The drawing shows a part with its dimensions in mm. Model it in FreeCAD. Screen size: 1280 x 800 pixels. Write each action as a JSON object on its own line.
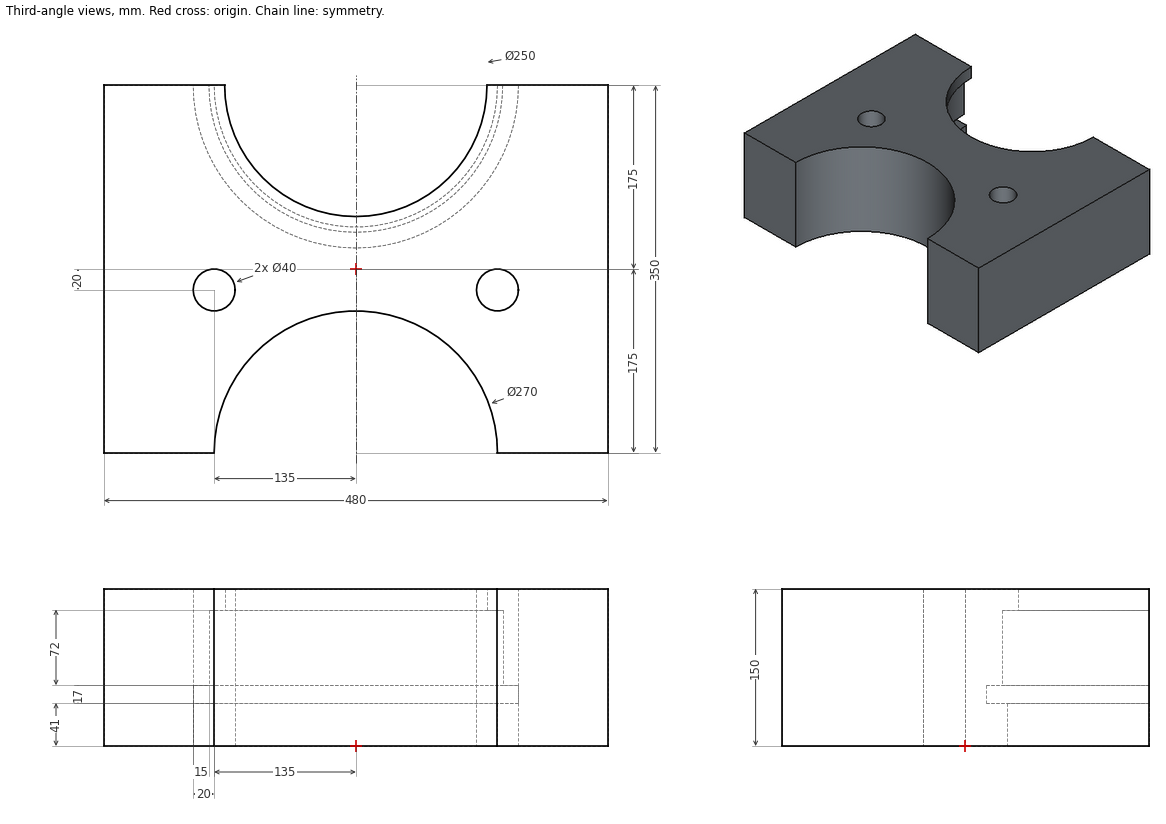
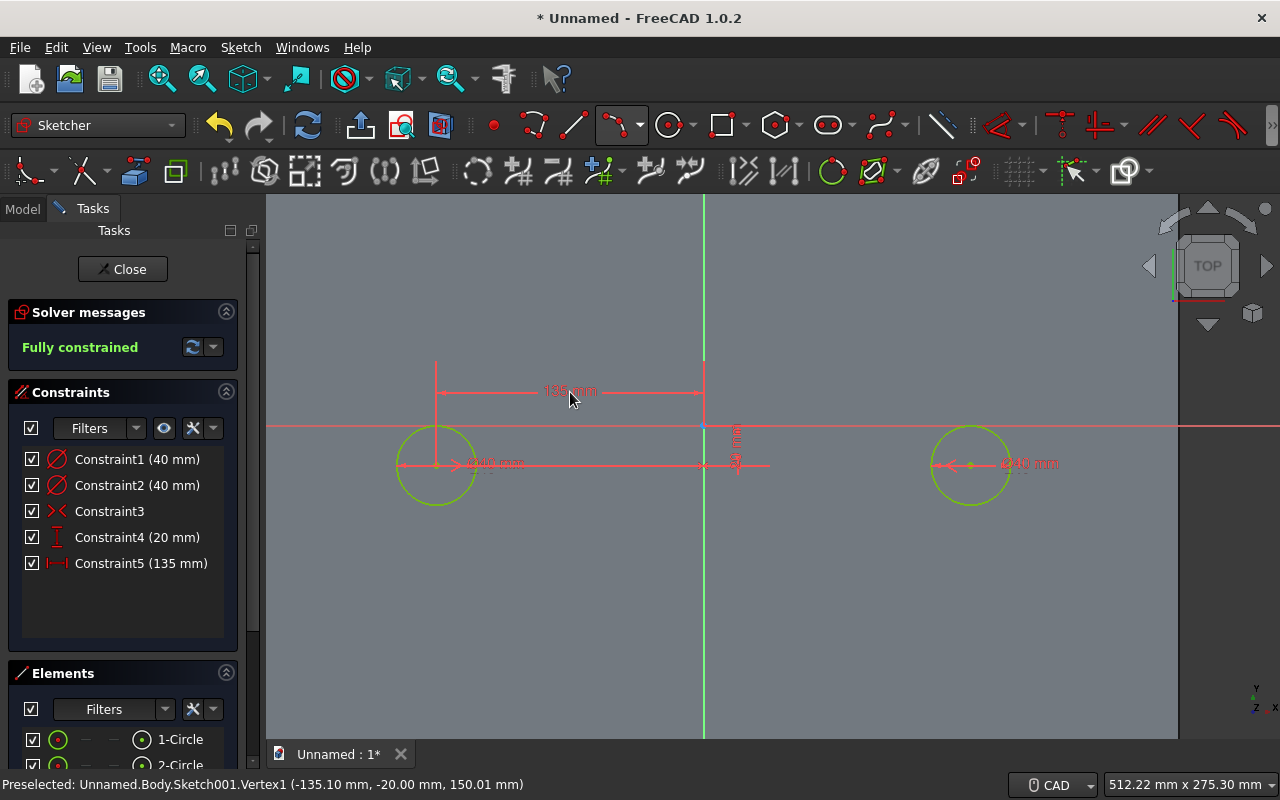
{"action": "left_click", "coordinate": [123, 269]}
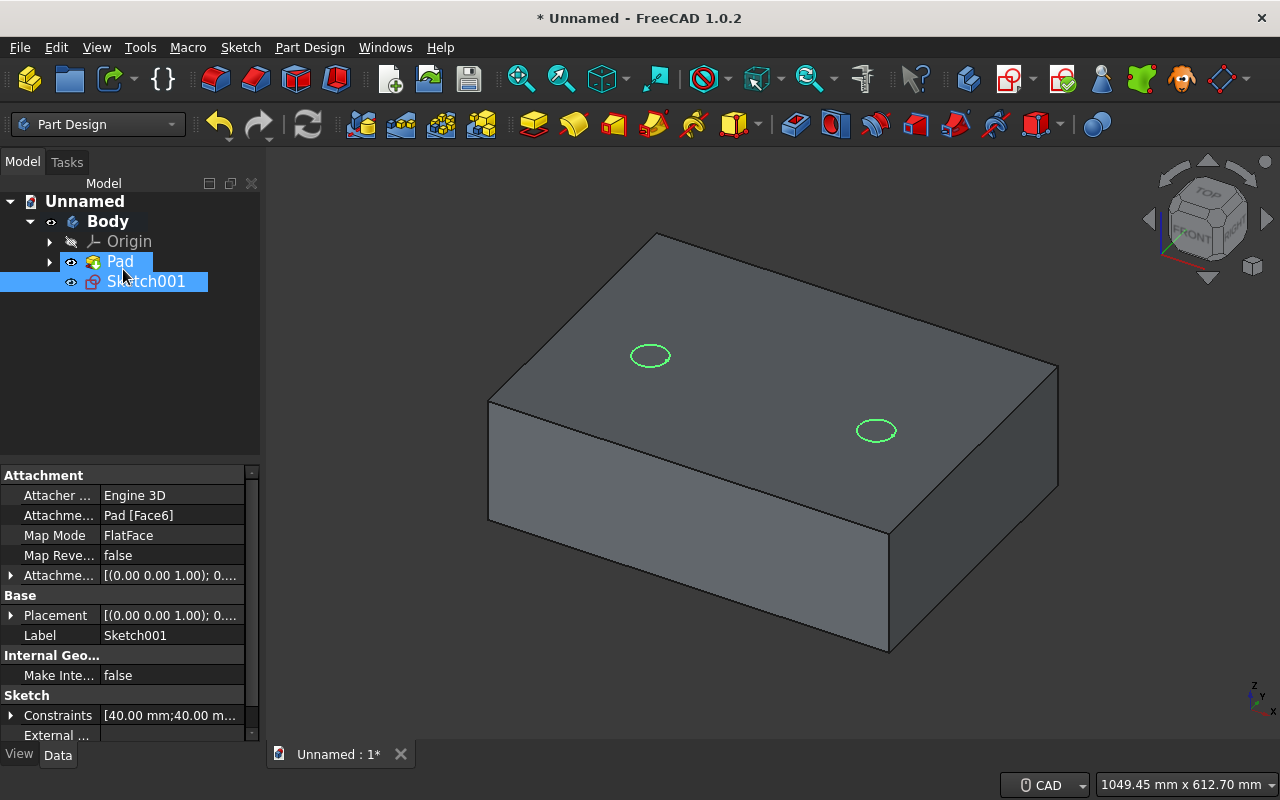
{"action": "left_click", "coordinate": [796, 124]}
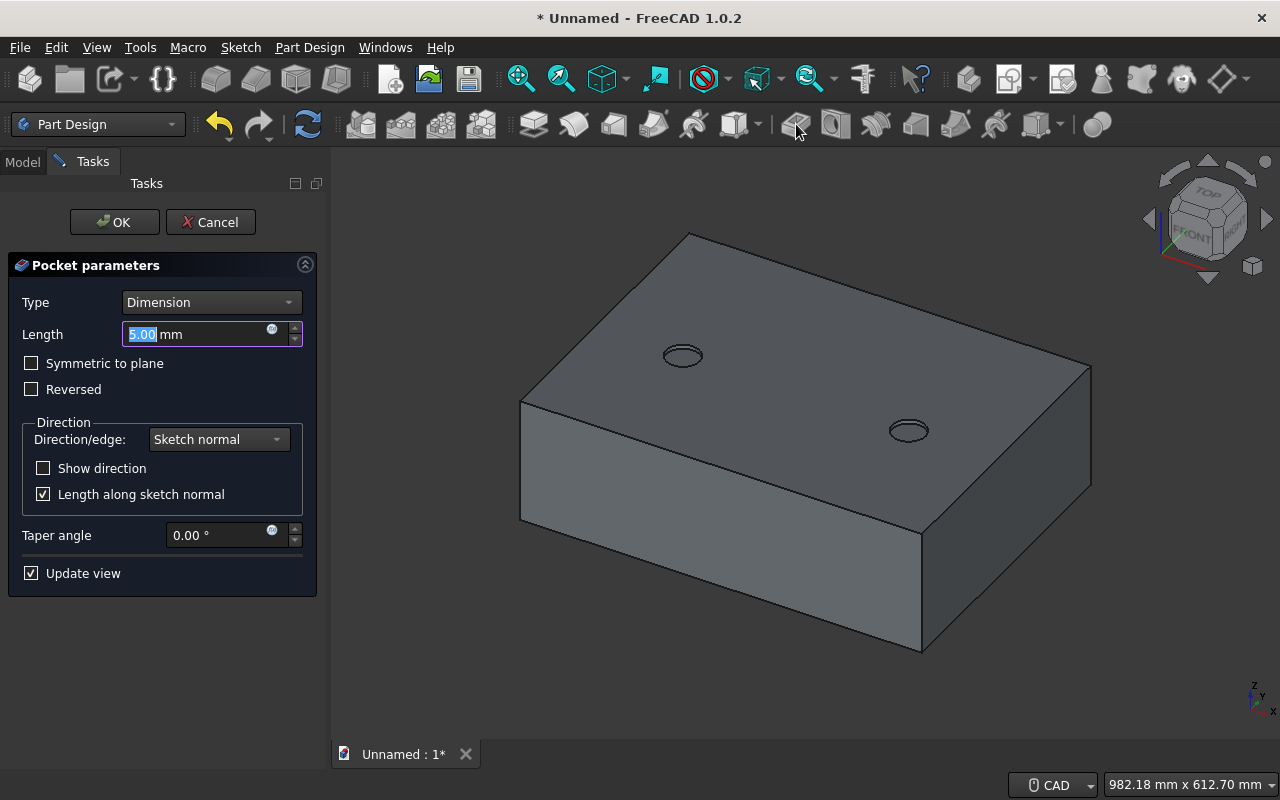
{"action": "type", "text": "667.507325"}
{"action": "key", "text": "Tab"}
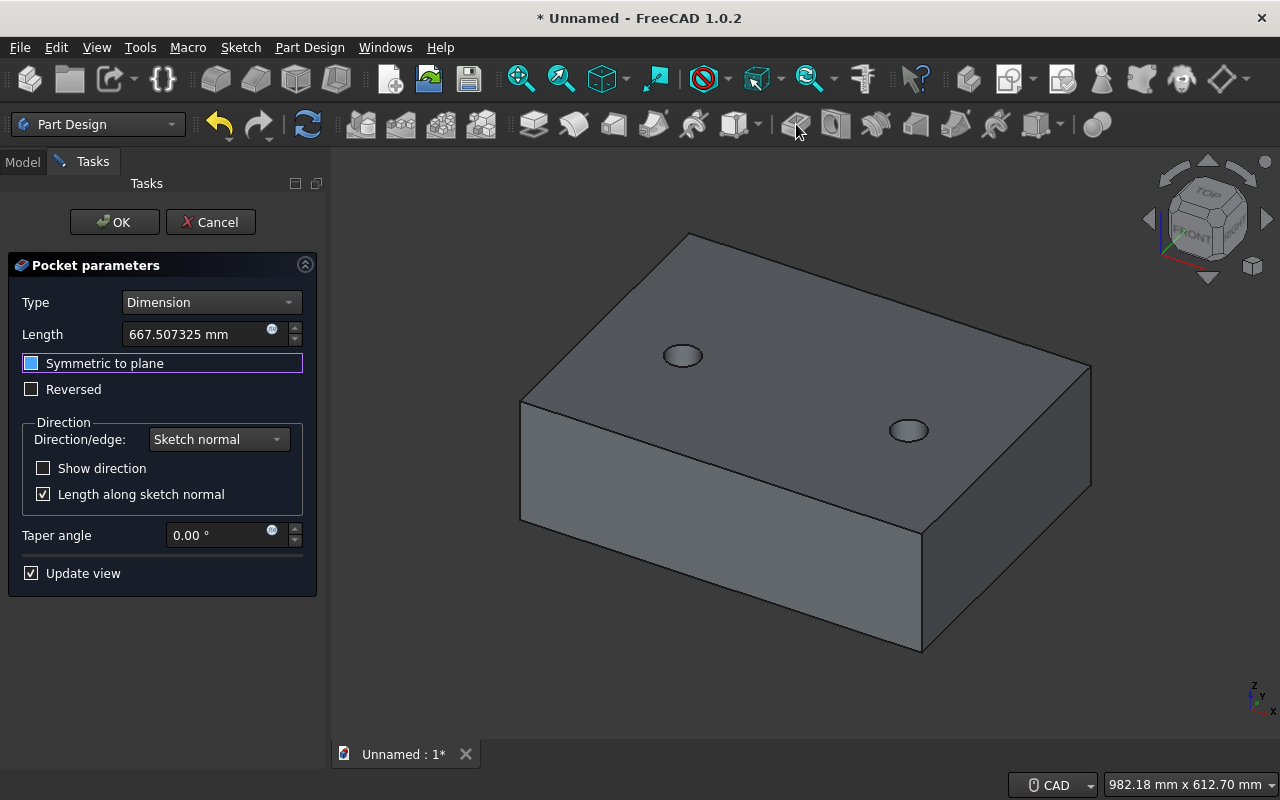
{"action": "left_click", "coordinate": [30, 363]}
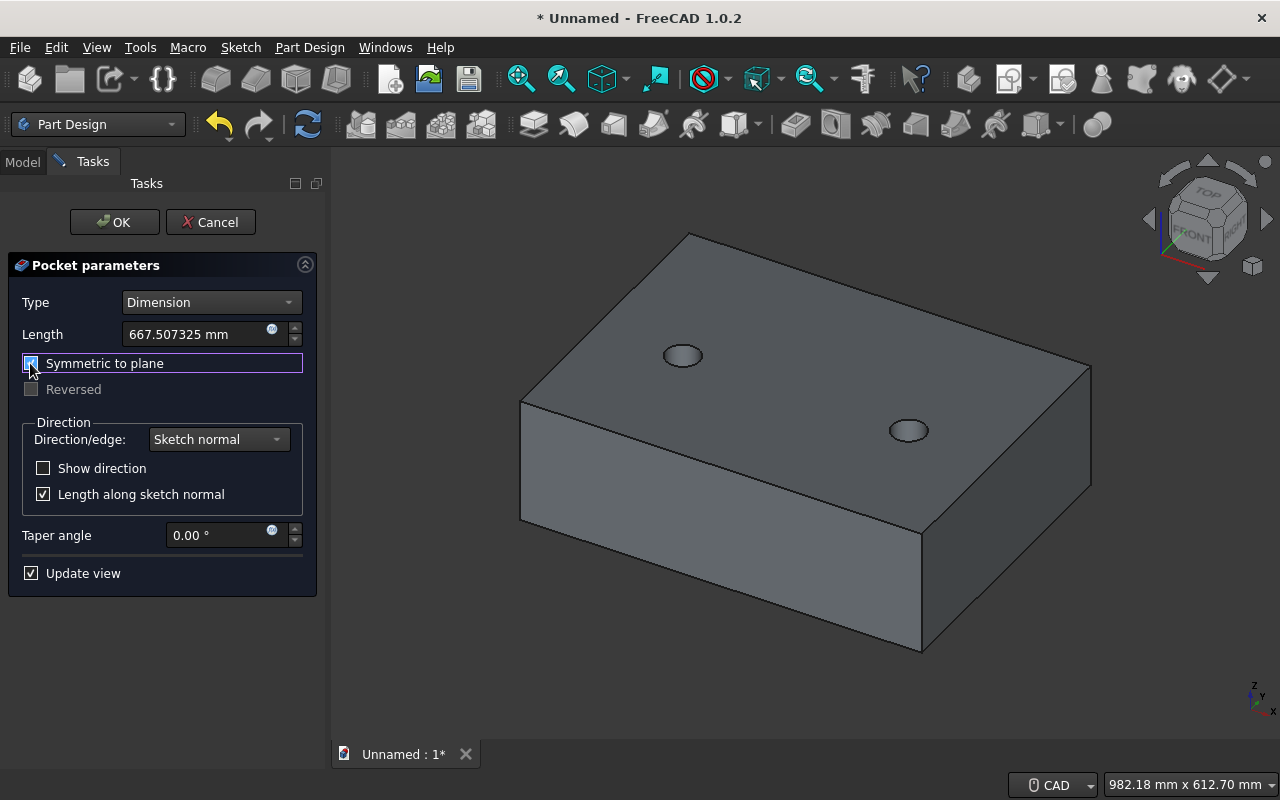
{"action": "left_click", "coordinate": [115, 222]}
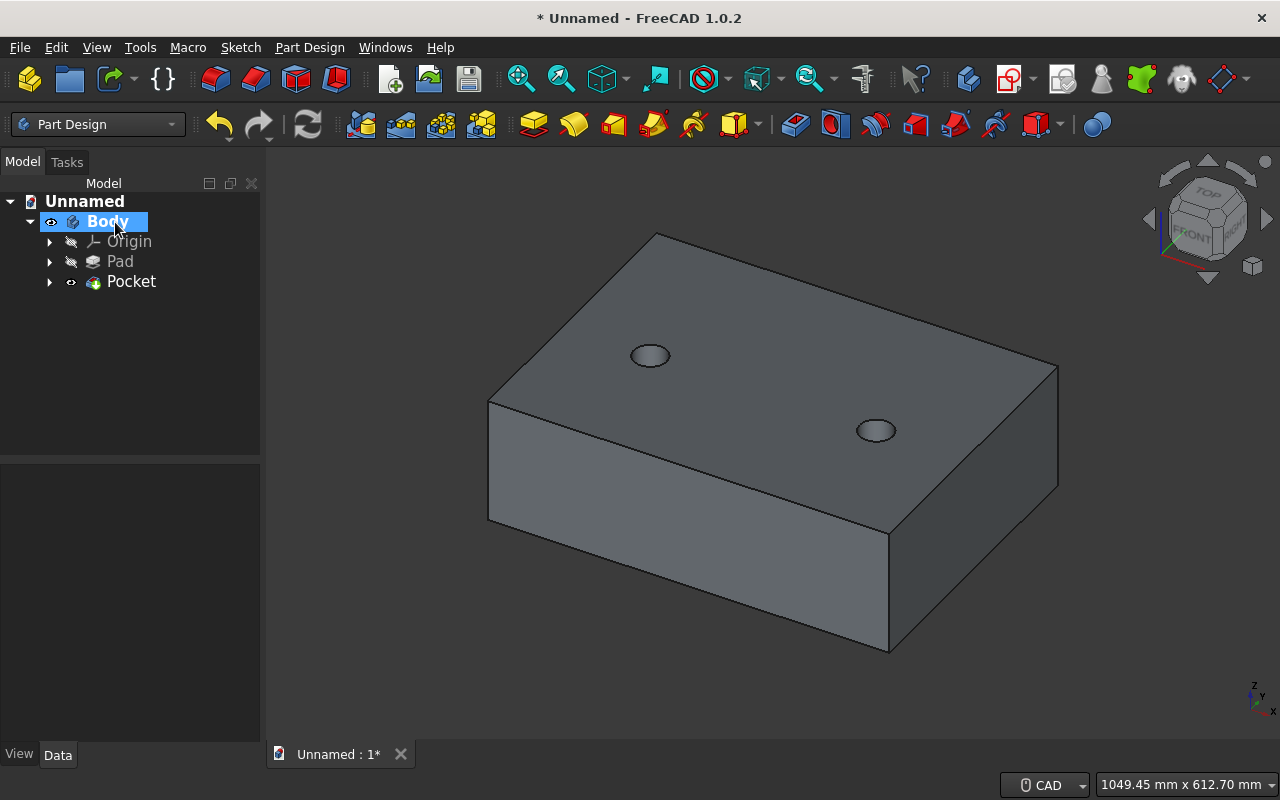
{"action": "left_click", "coordinate": [797, 359]}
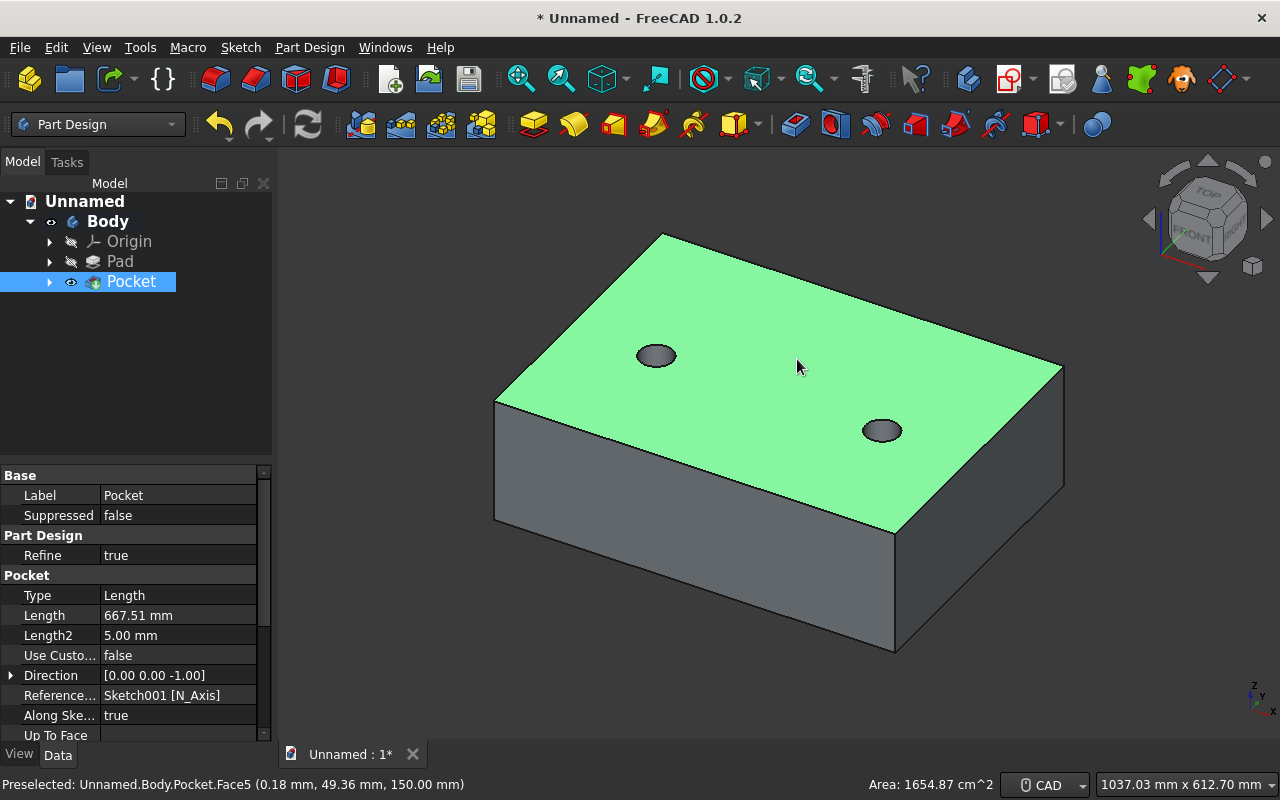
{"action": "left_click", "coordinate": [1010, 80]}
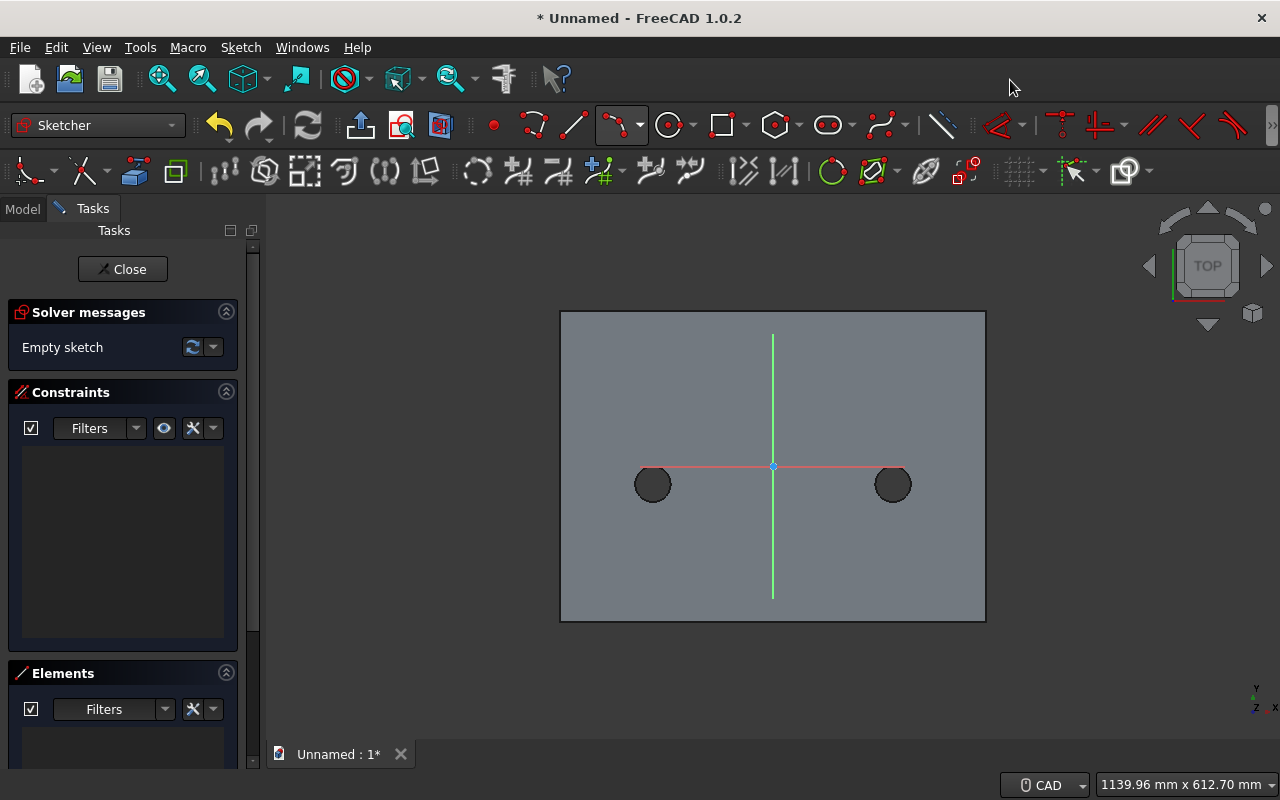
{"action": "scroll", "coordinate": [565, 457], "scroll_direction": "down", "scroll_amount": 2}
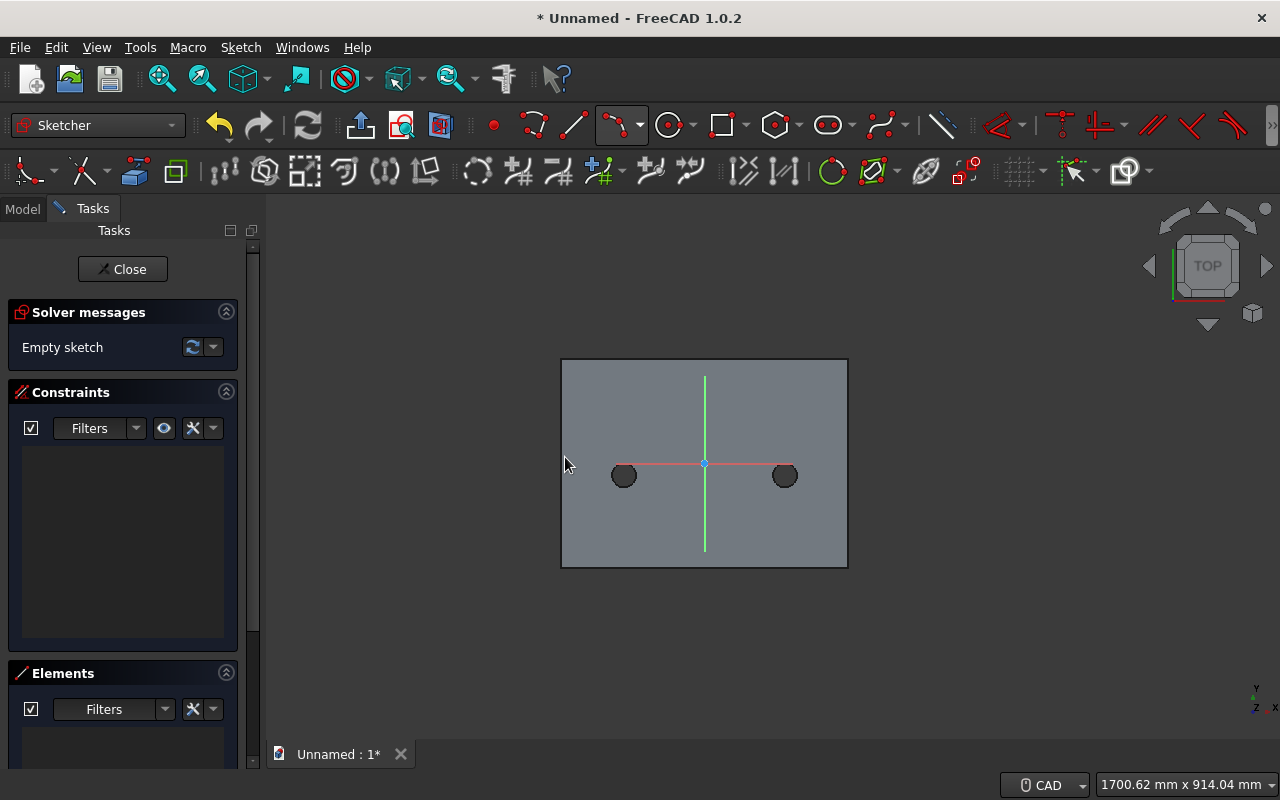
{"action": "key", "text": "g c"}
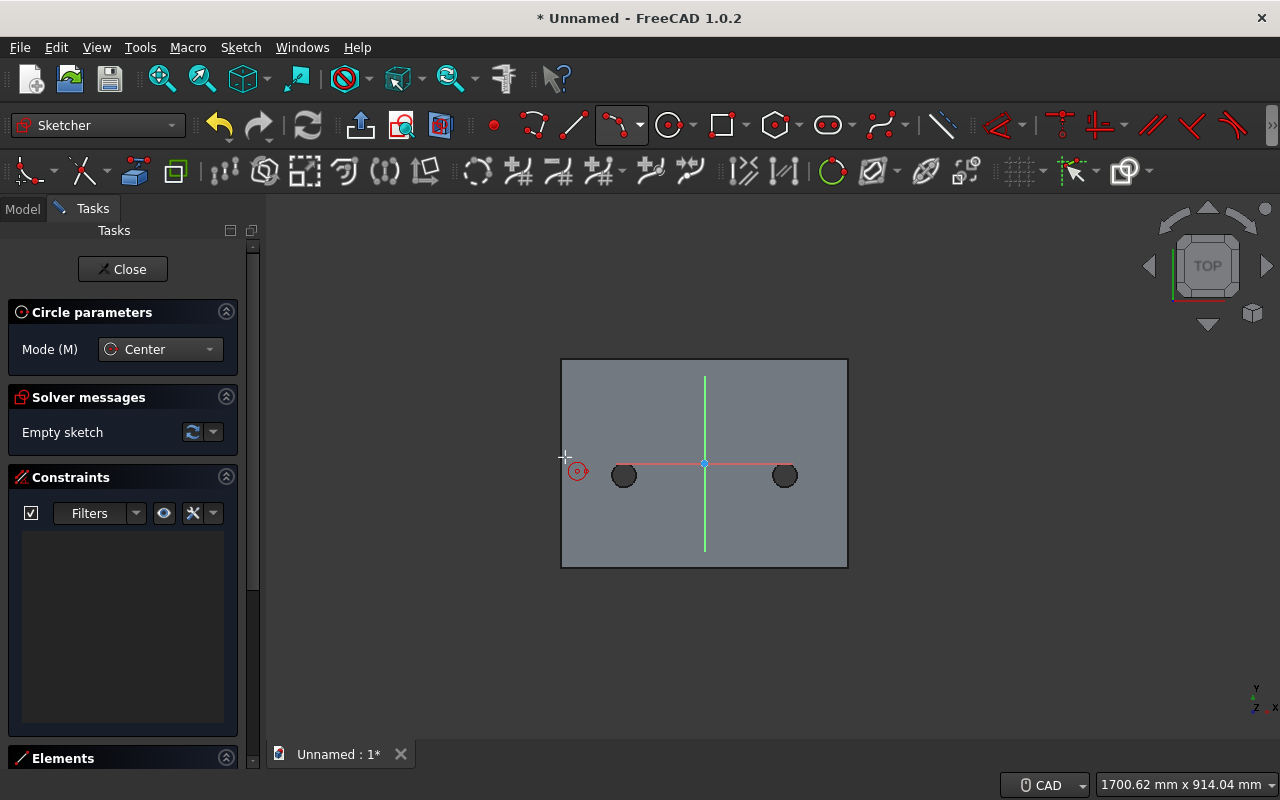
{"action": "left_click", "coordinate": [705, 568]}
{"action": "mouse_move", "coordinate": [761, 511]}